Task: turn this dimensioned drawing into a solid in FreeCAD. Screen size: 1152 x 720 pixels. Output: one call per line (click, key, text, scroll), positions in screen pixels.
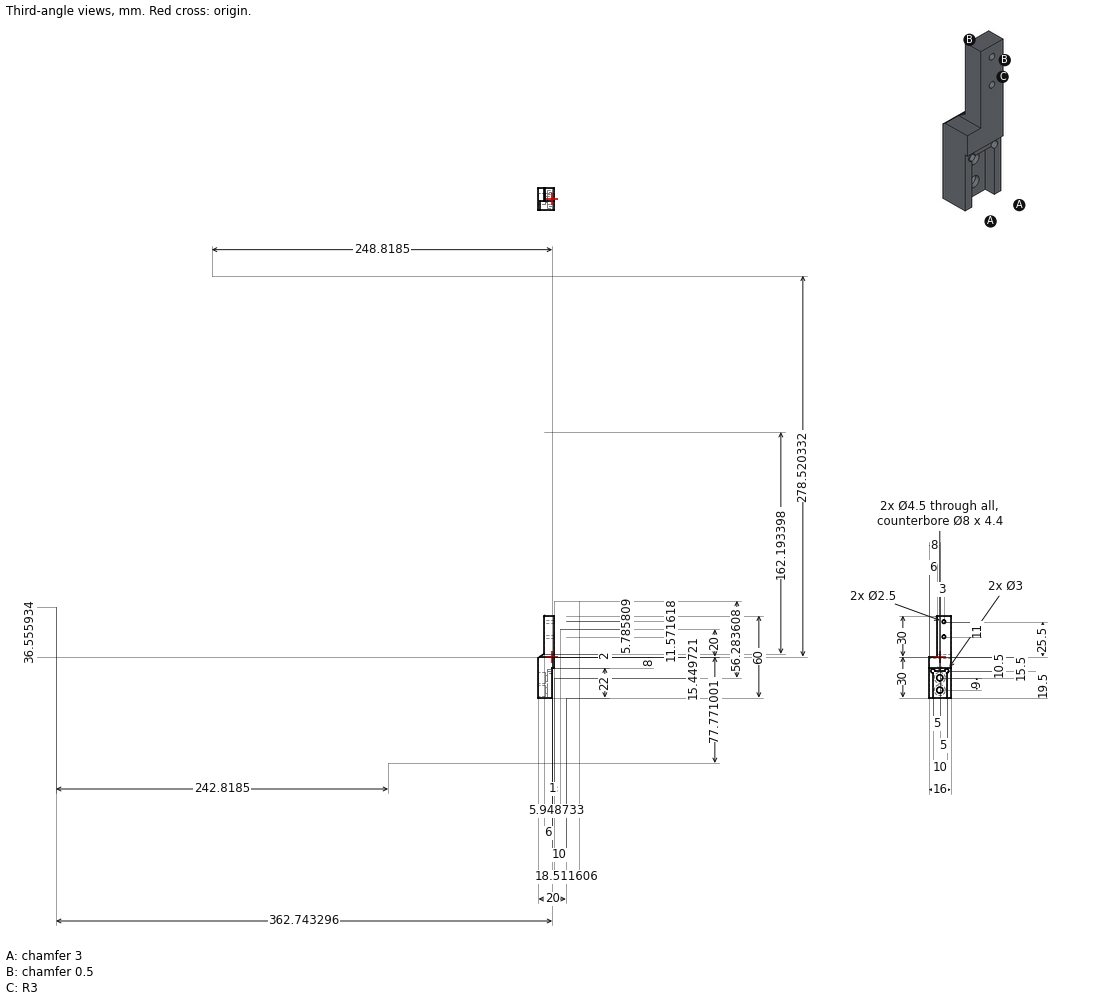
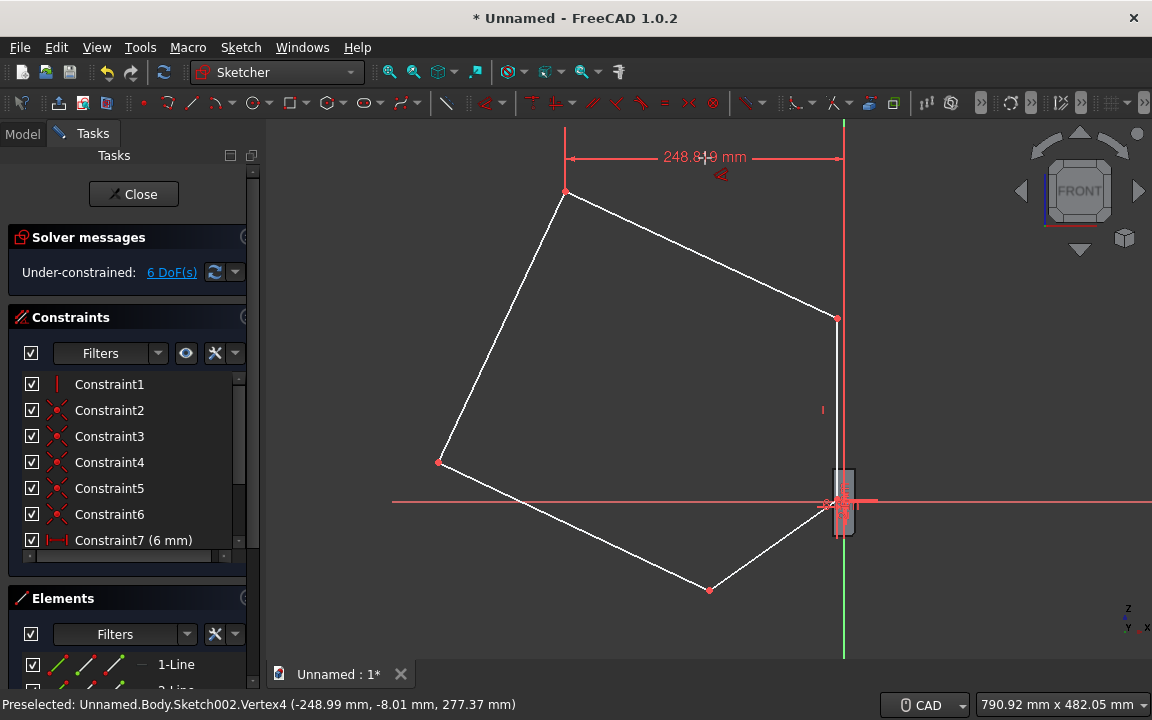
click(520, 501)
click(574, 625)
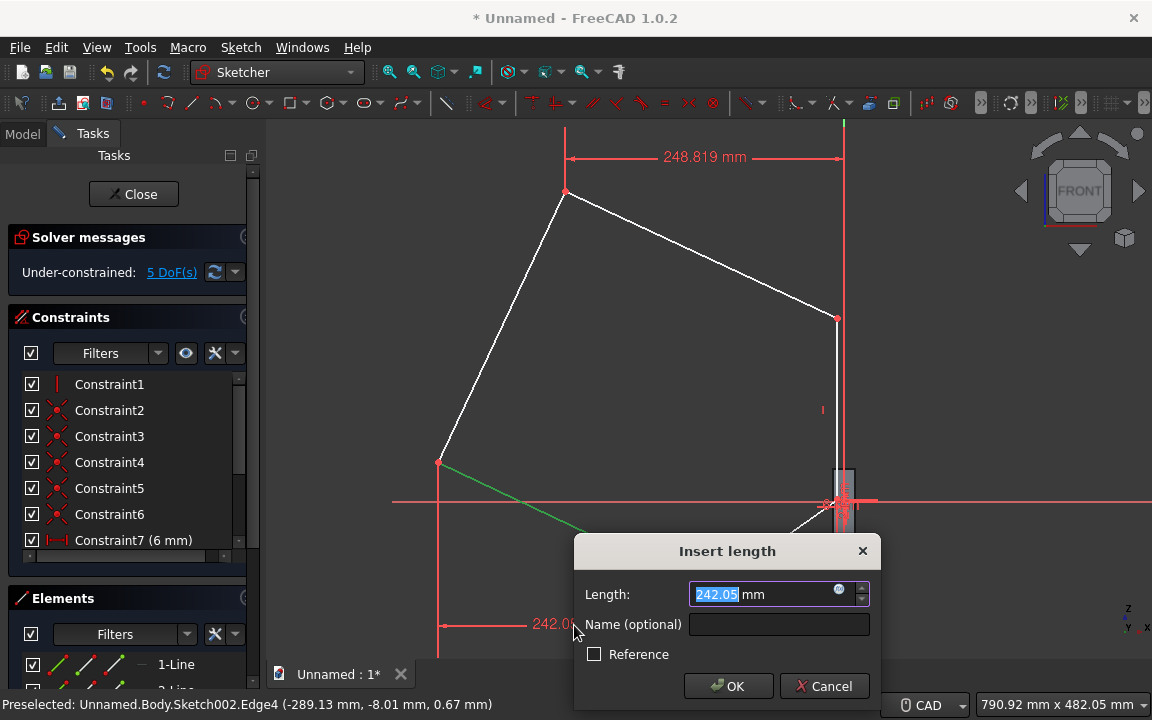
text(242.8185)
key(Return)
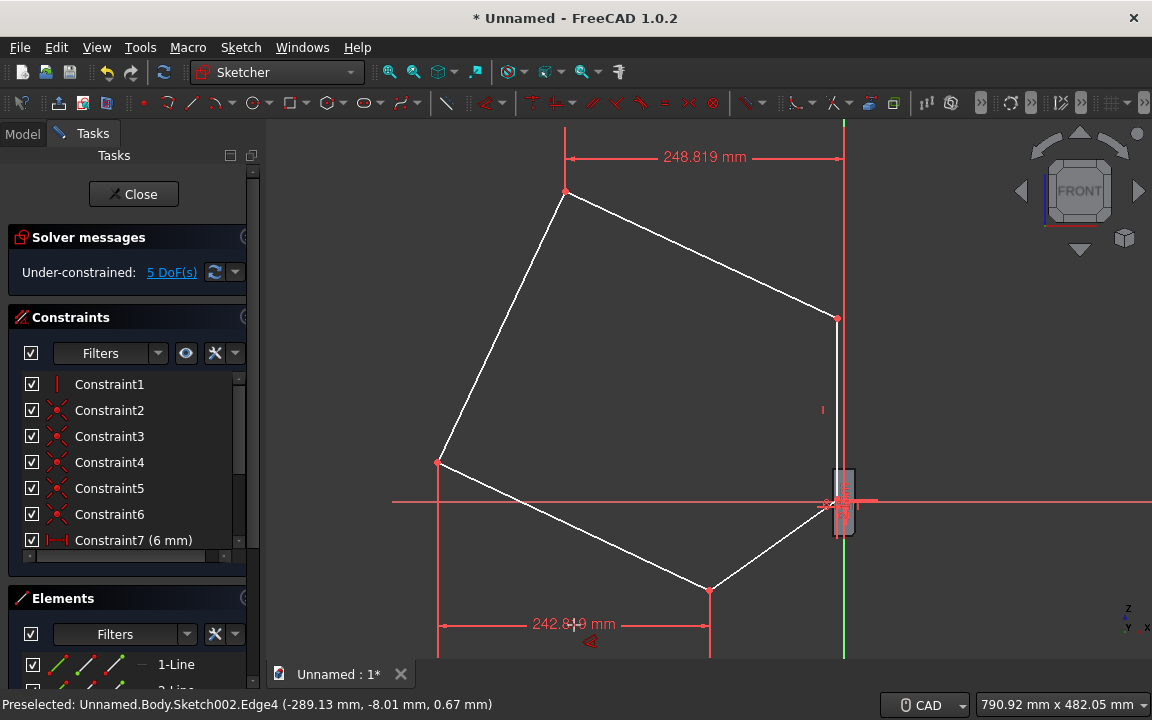
scroll(837, 446, up, 4)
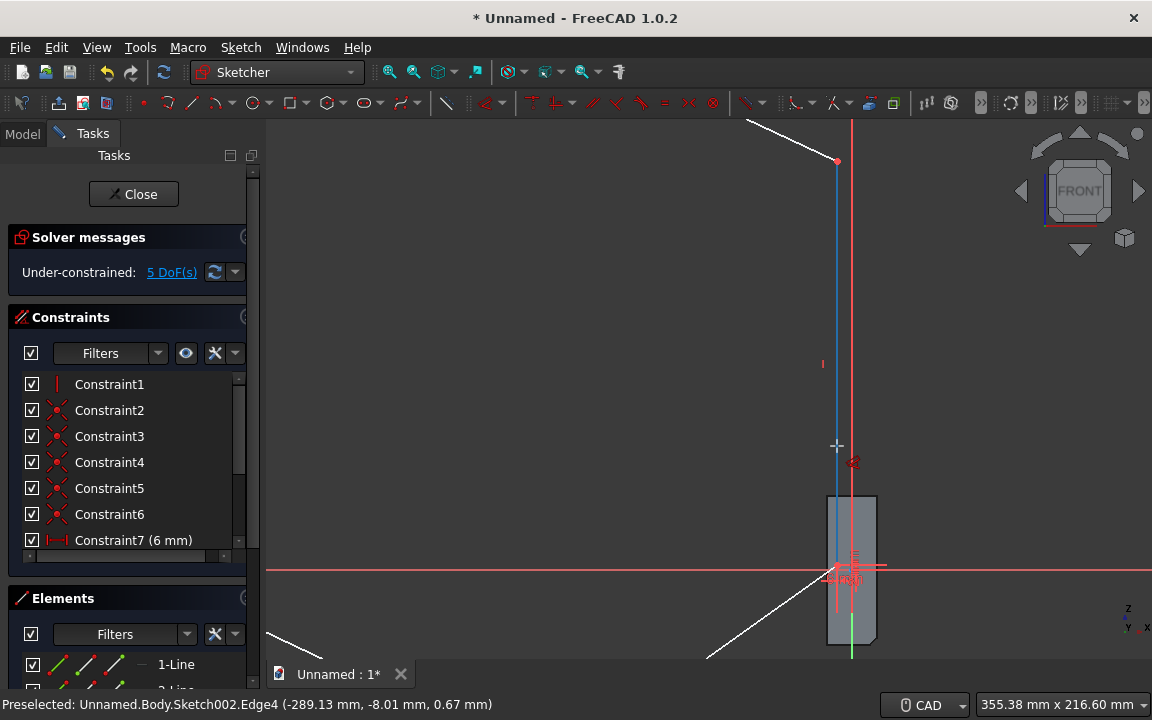
click(837, 444)
click(871, 363)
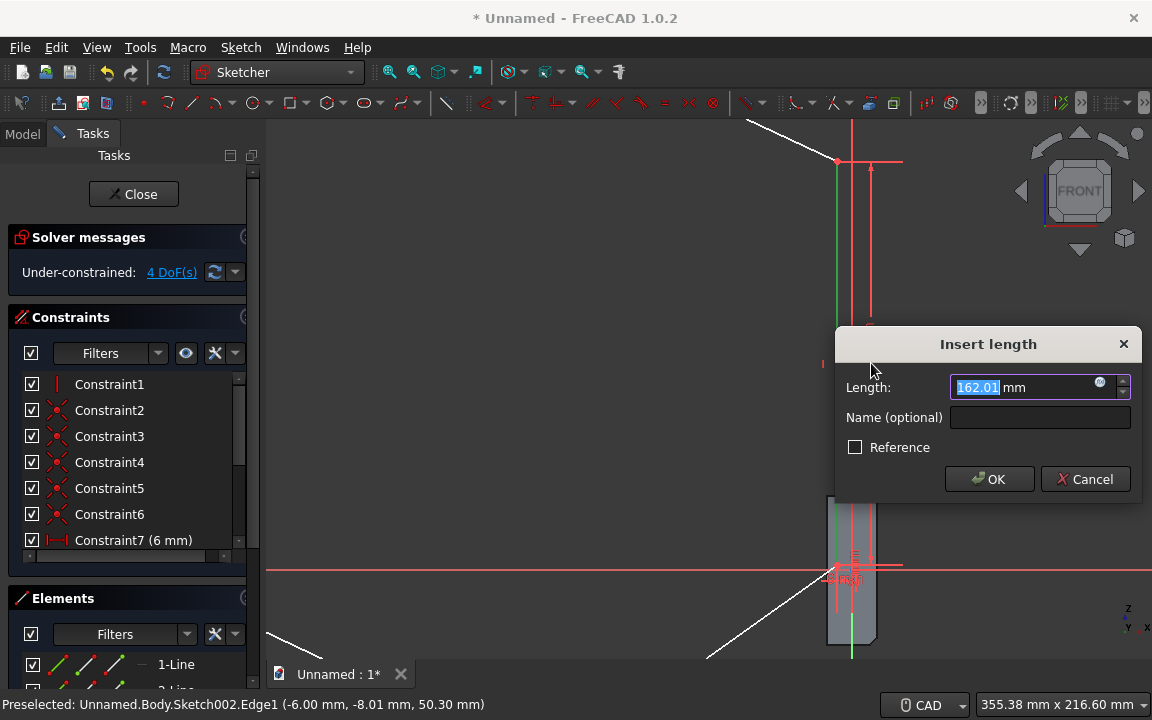
text(162.193398)
key(Return)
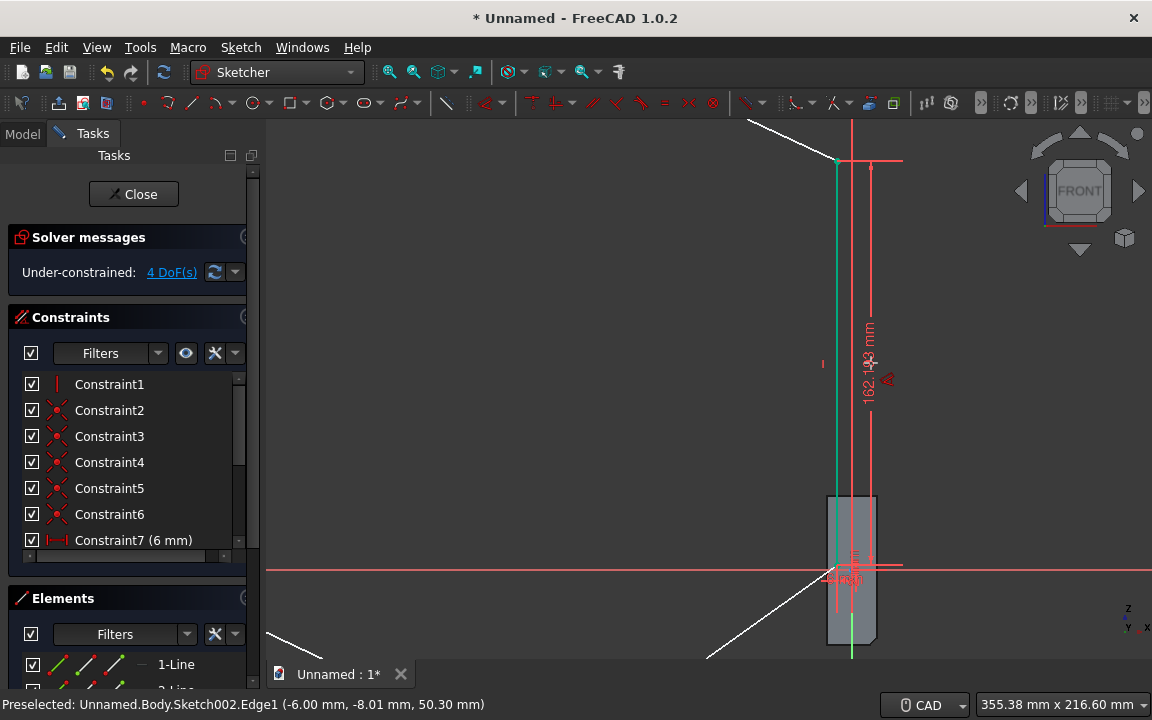
scroll(781, 429, down, 5)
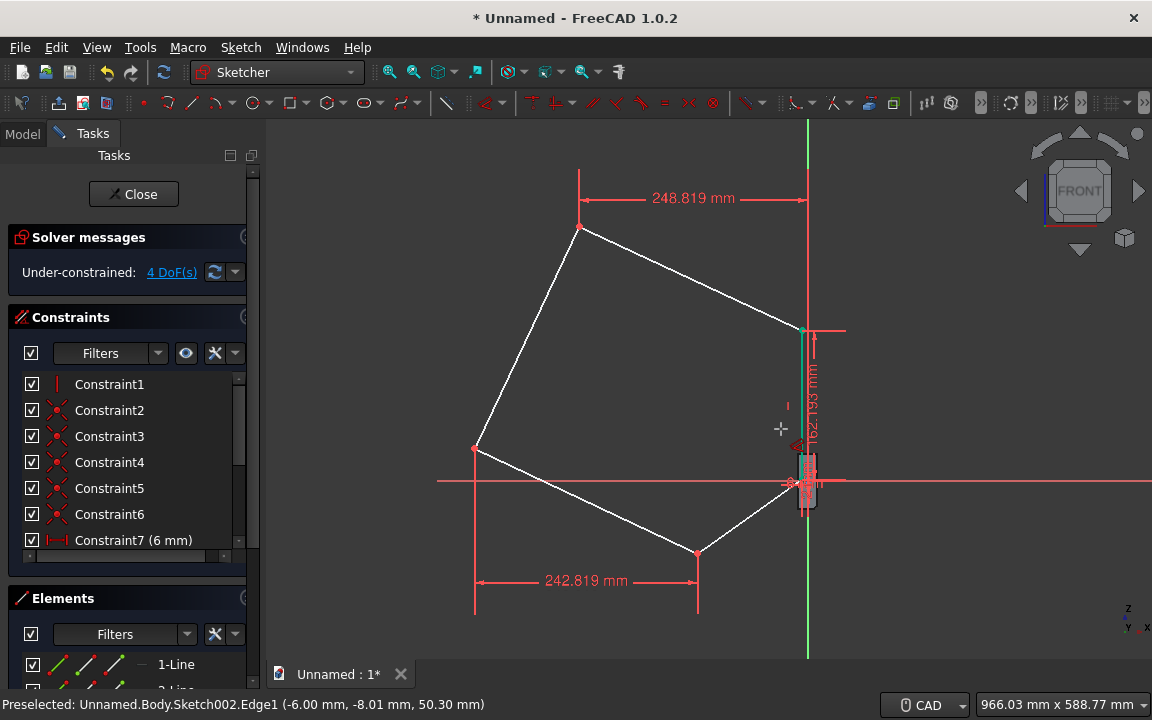
click(475, 449)
click(842, 458)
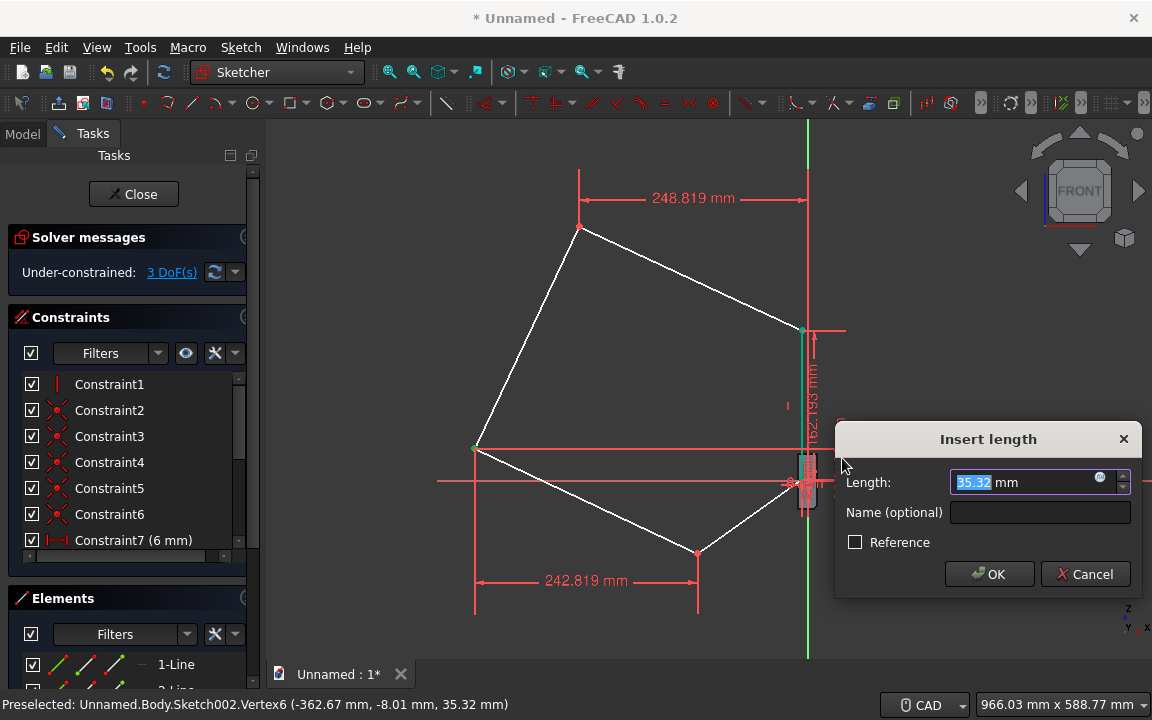
text(36.555934)
key(Return)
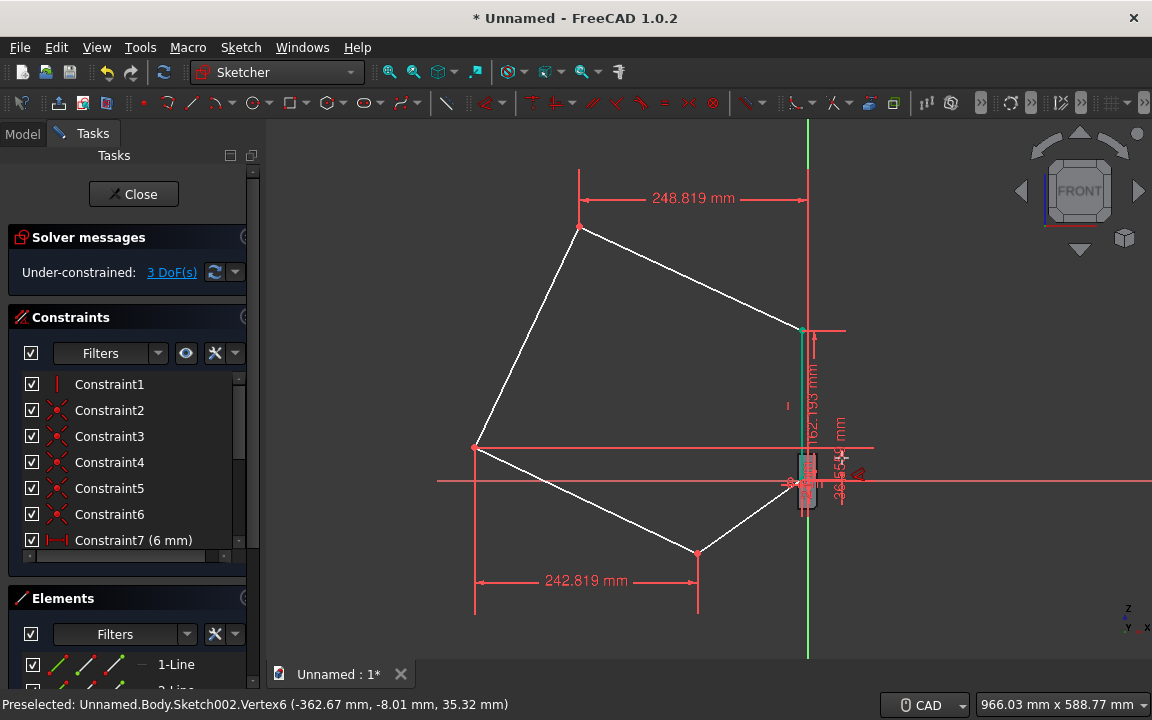
click(698, 554)
click(842, 518)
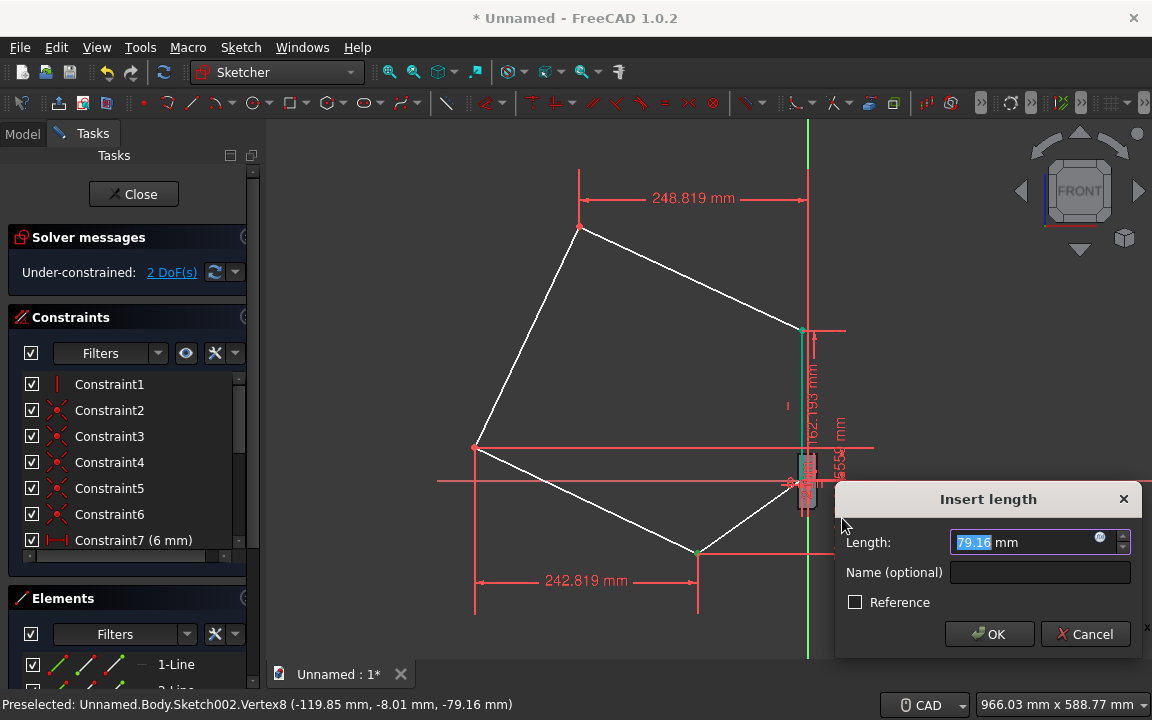
text(77.771001)
key(Return)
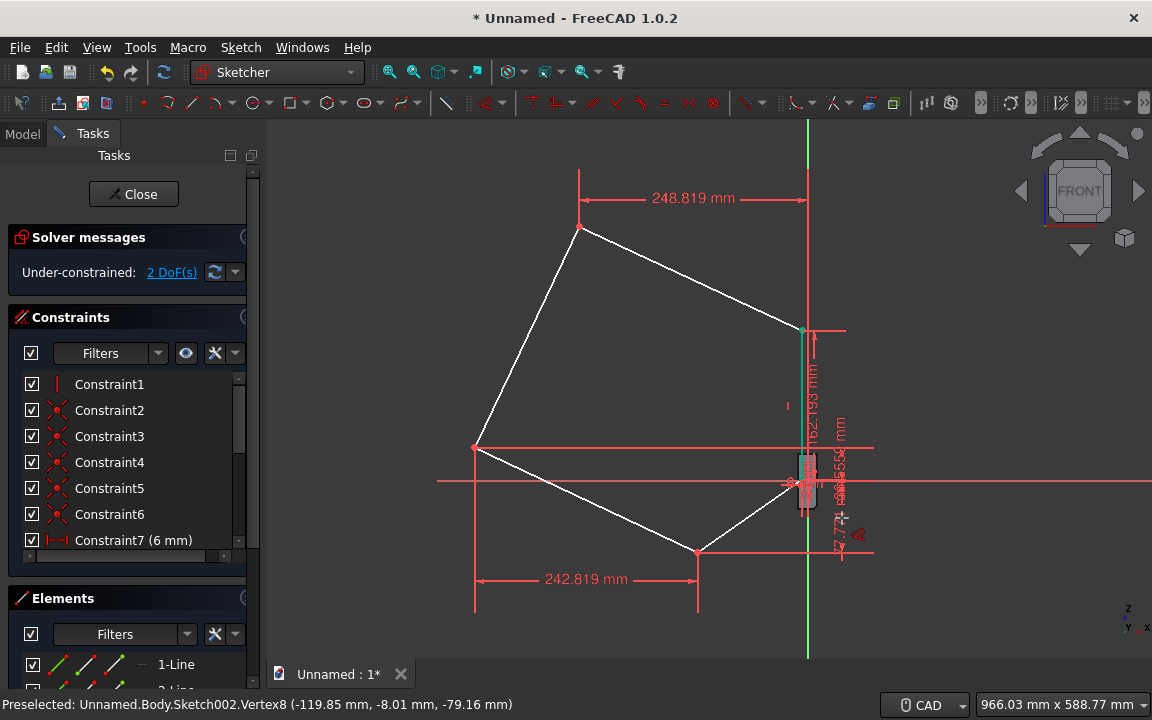
click(579, 227)
click(842, 354)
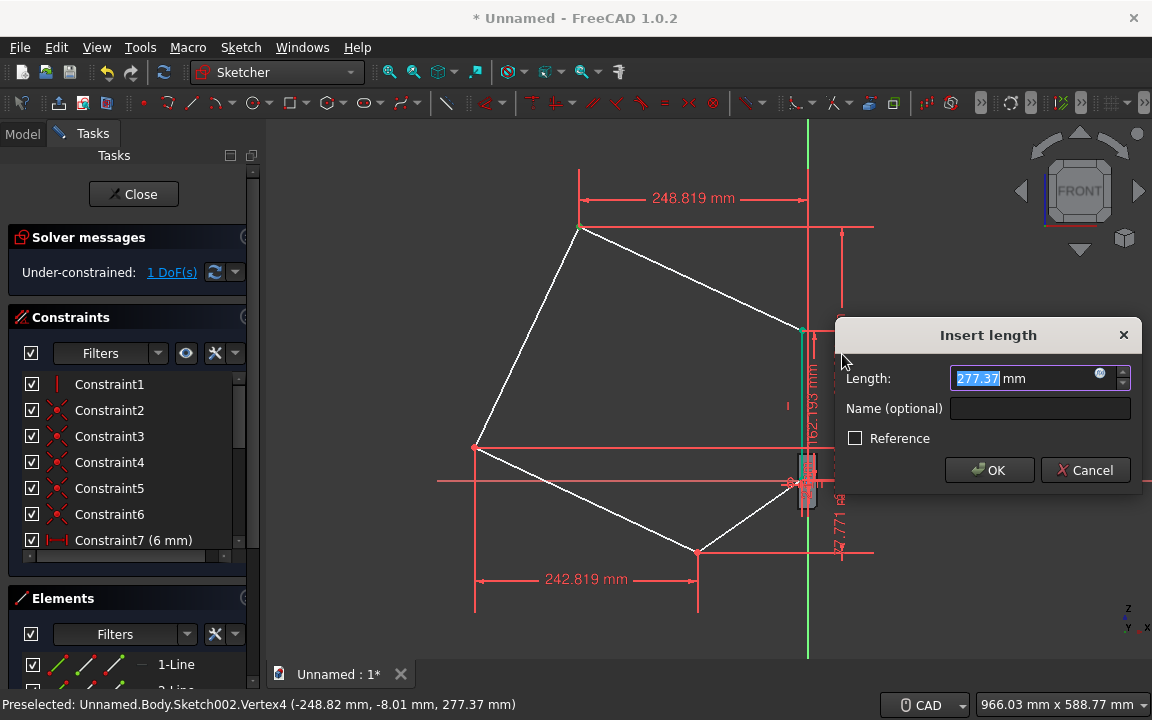
text(278.520332)
key(Return)